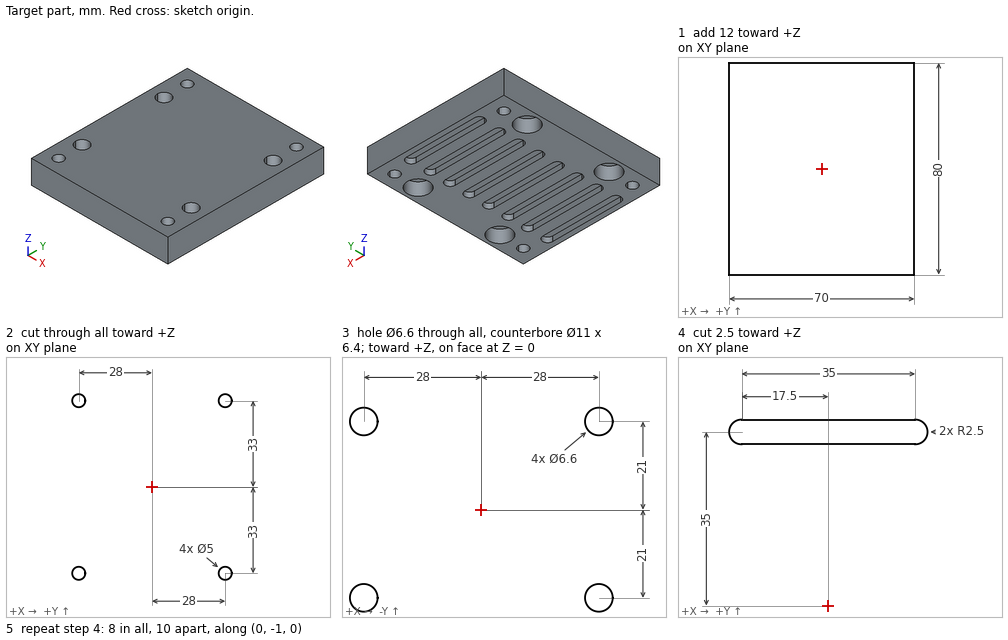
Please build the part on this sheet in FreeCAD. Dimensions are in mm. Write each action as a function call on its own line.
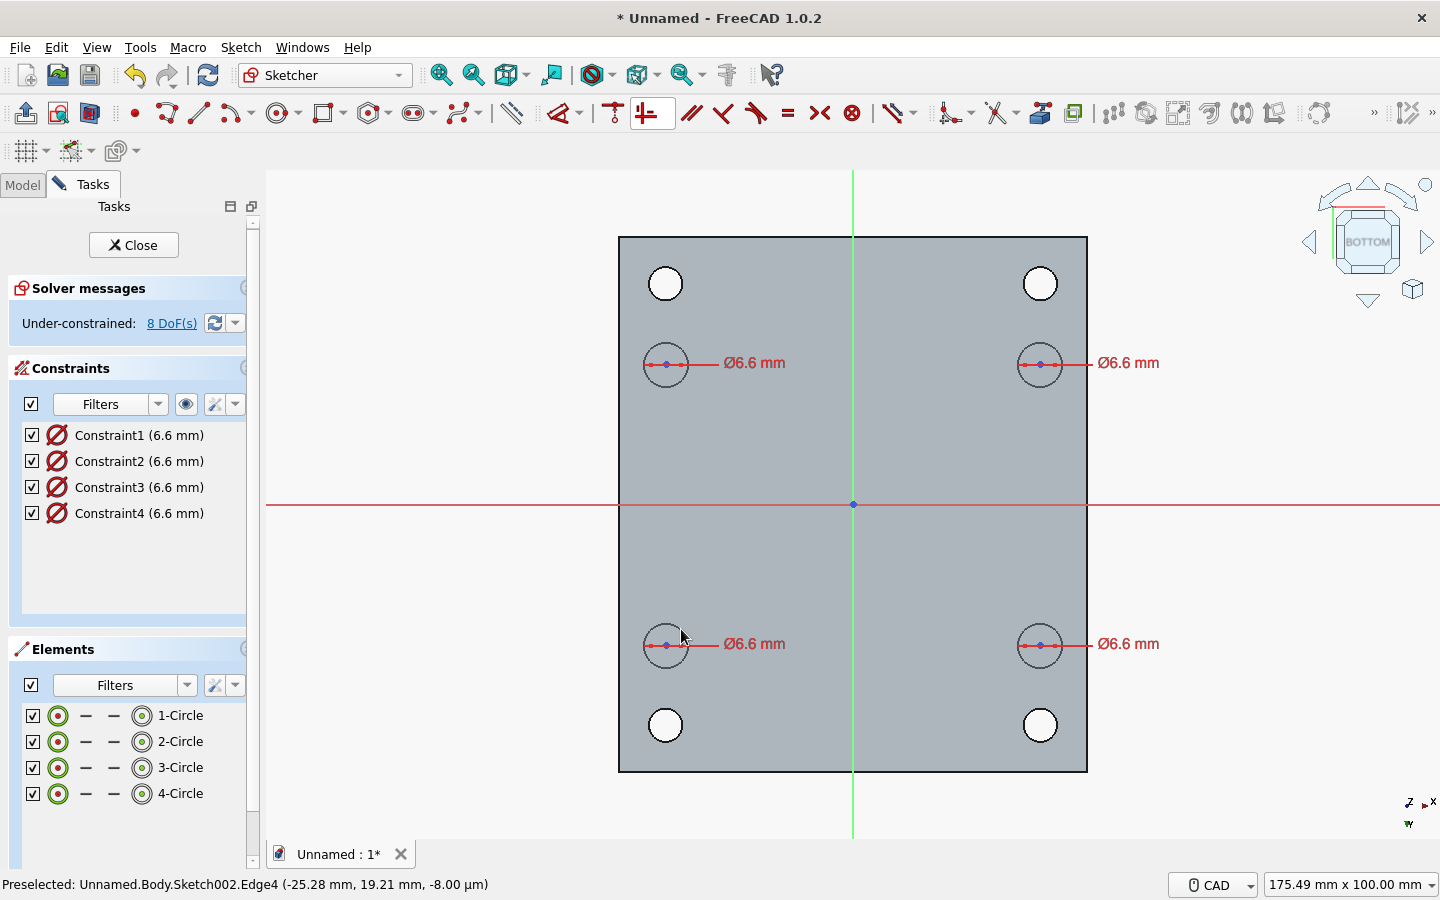
click(1040, 365)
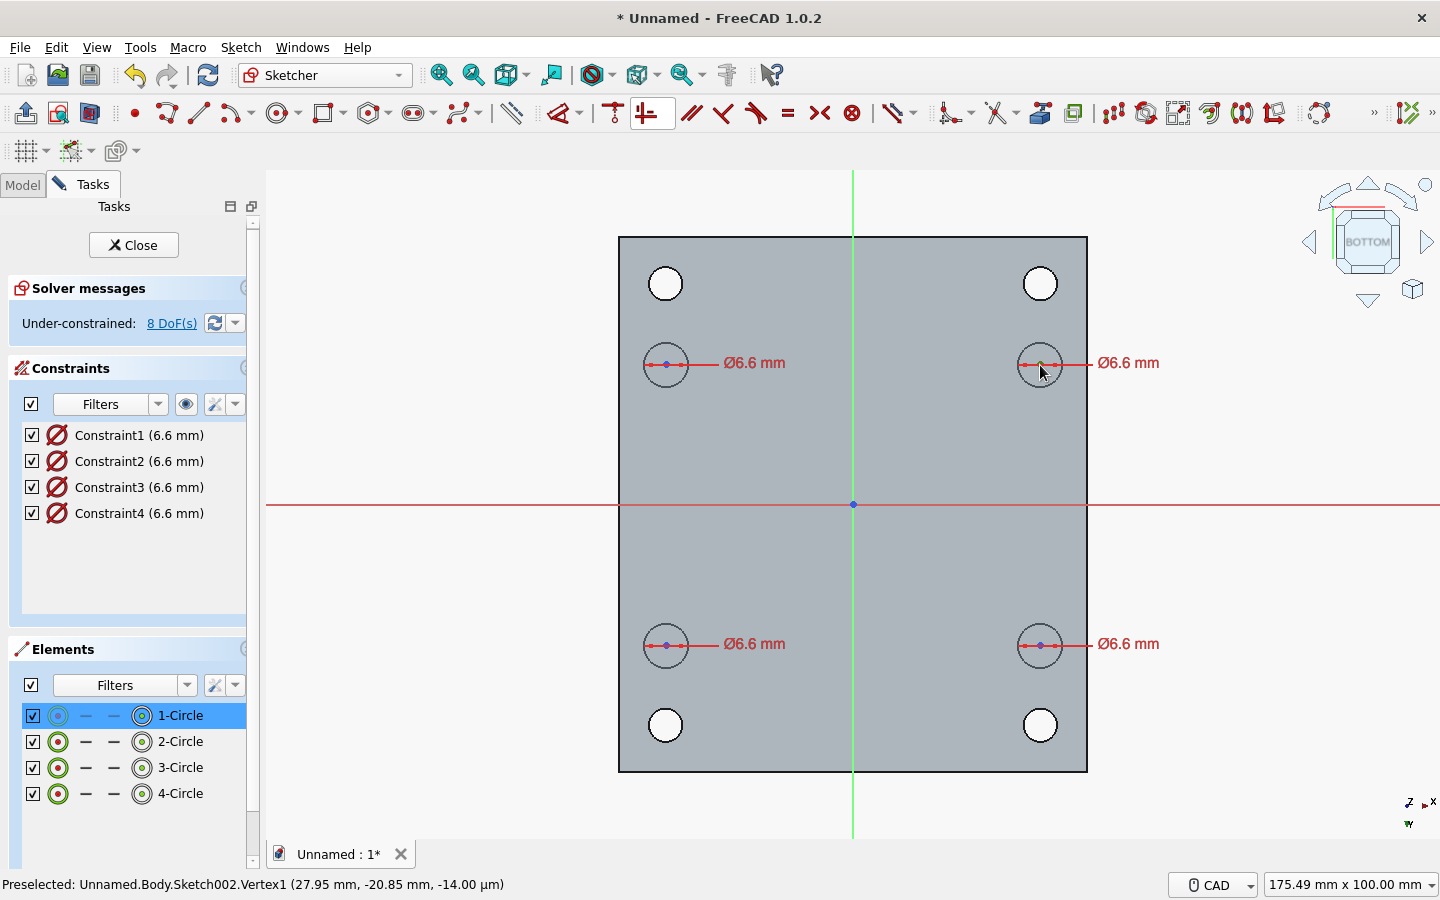
click(1040, 646)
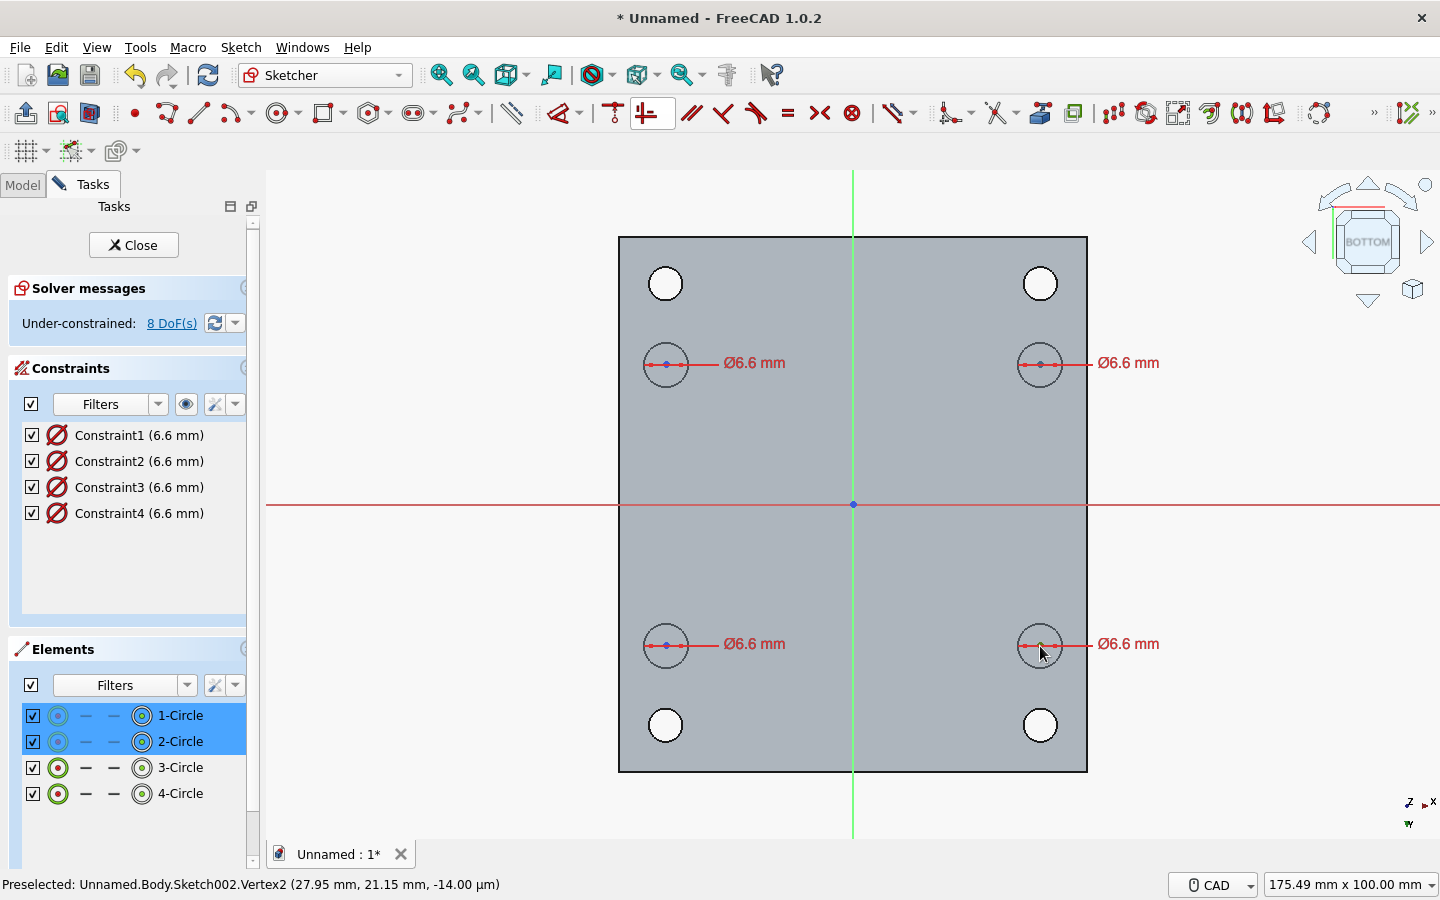
key(v)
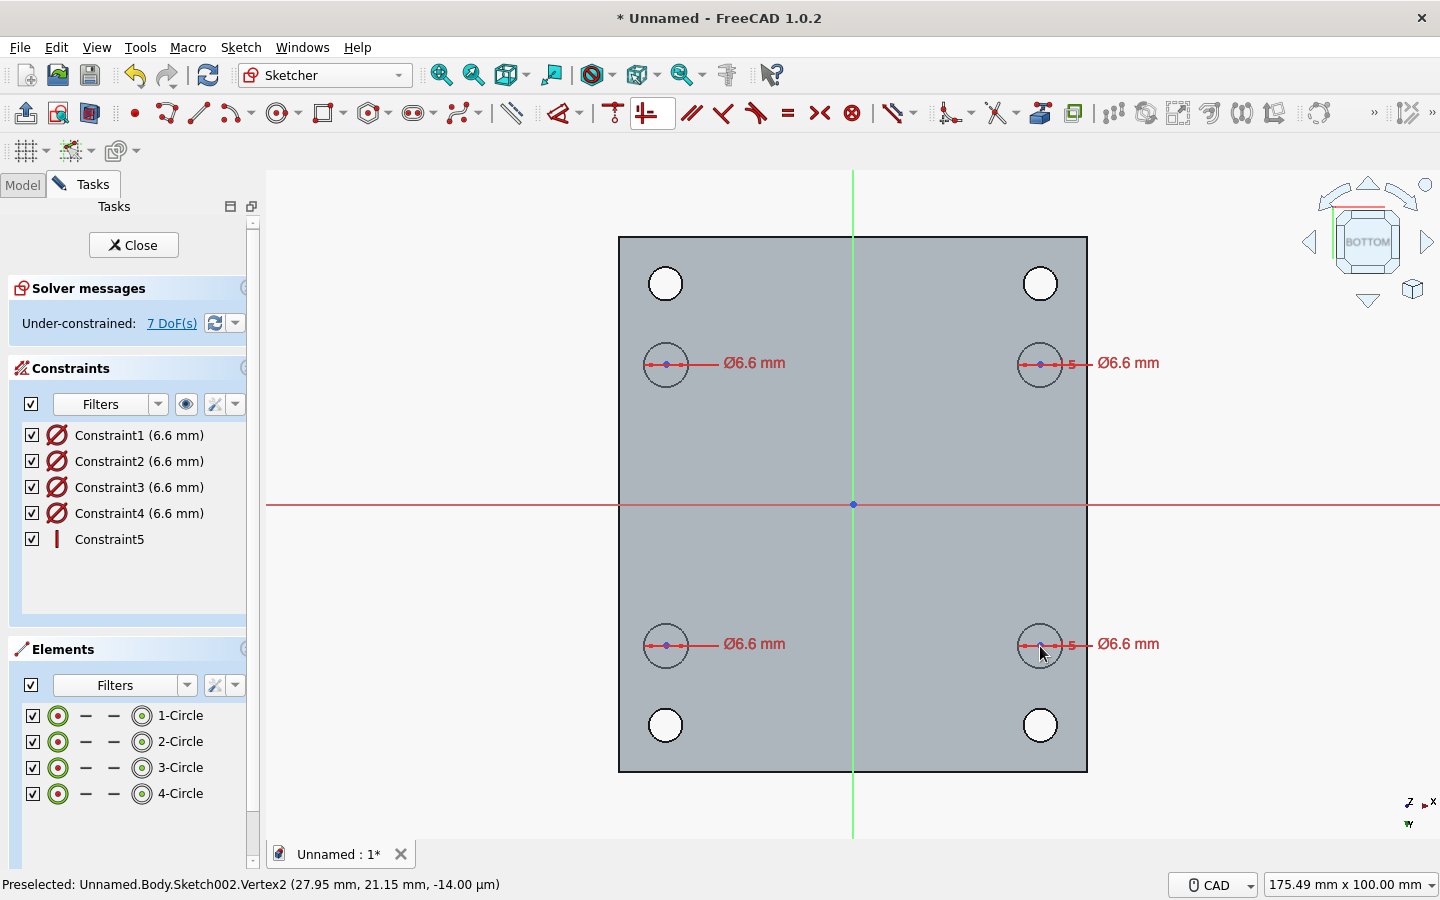
click(1040, 365)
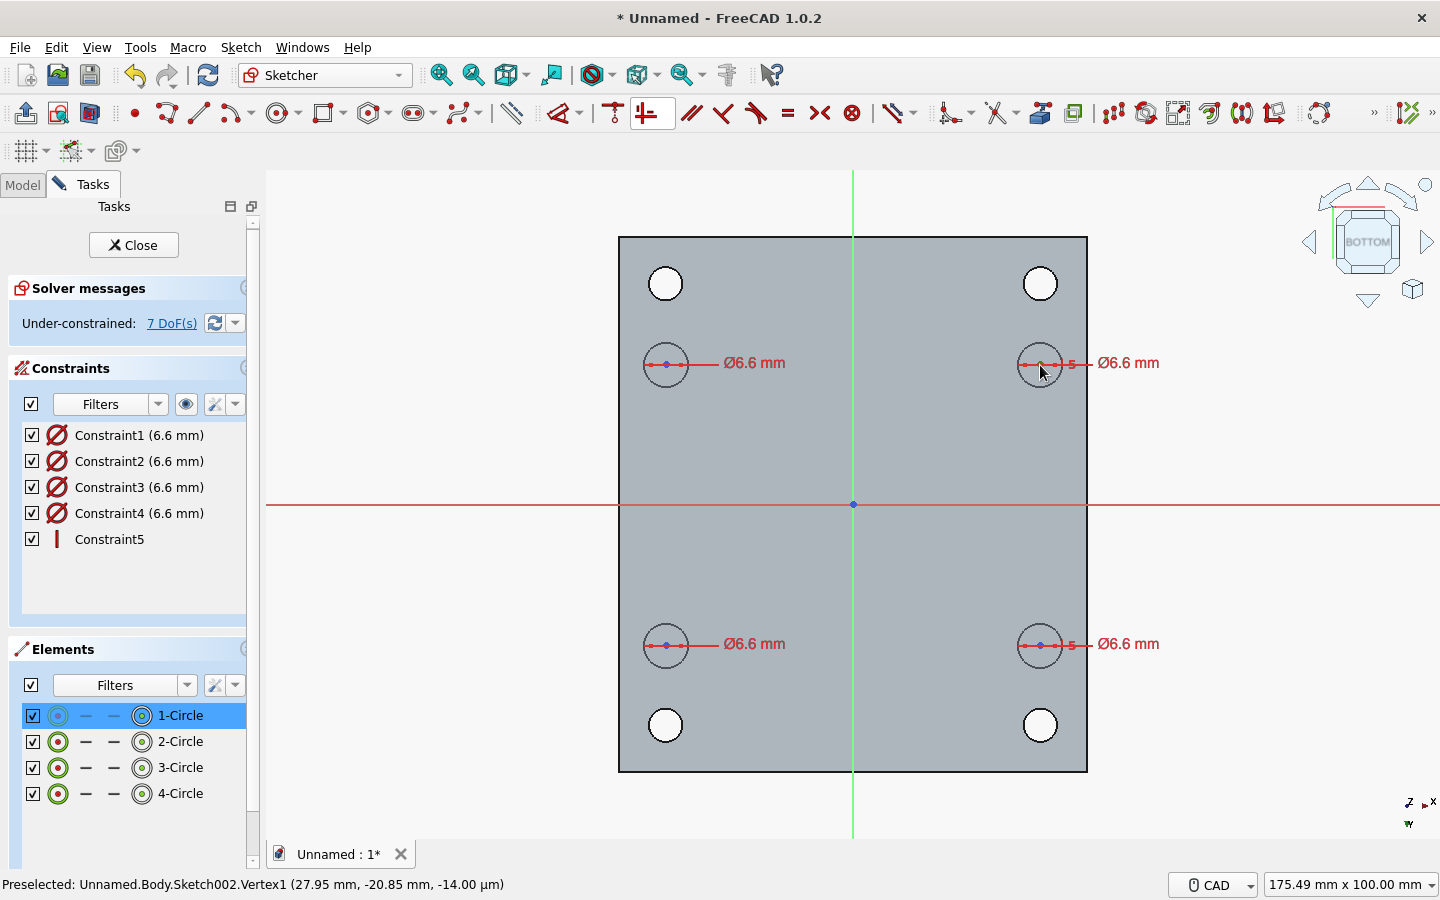
click(666, 365)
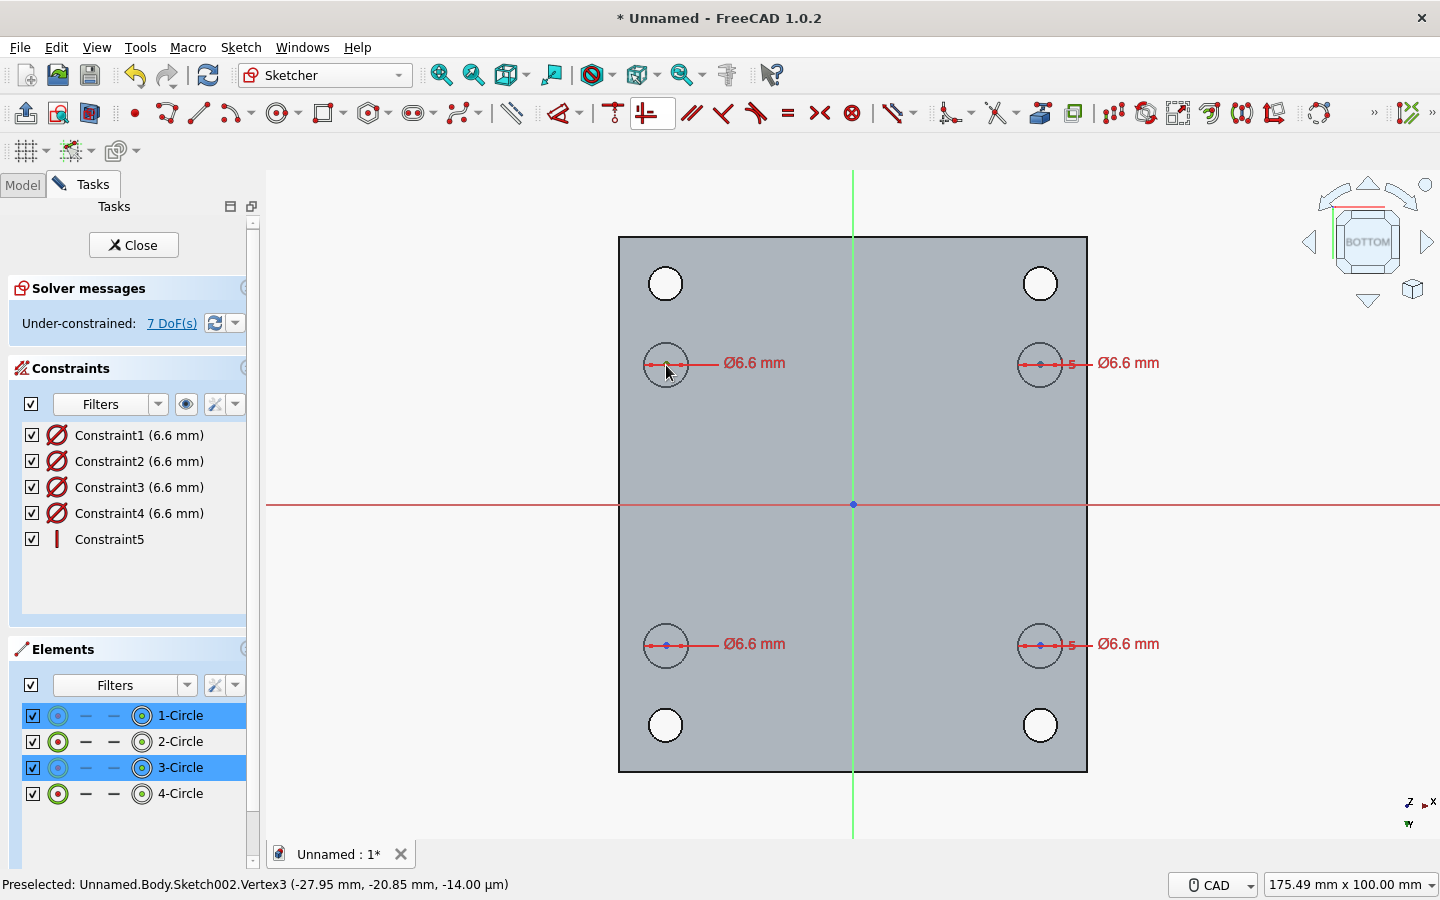
click(670, 114)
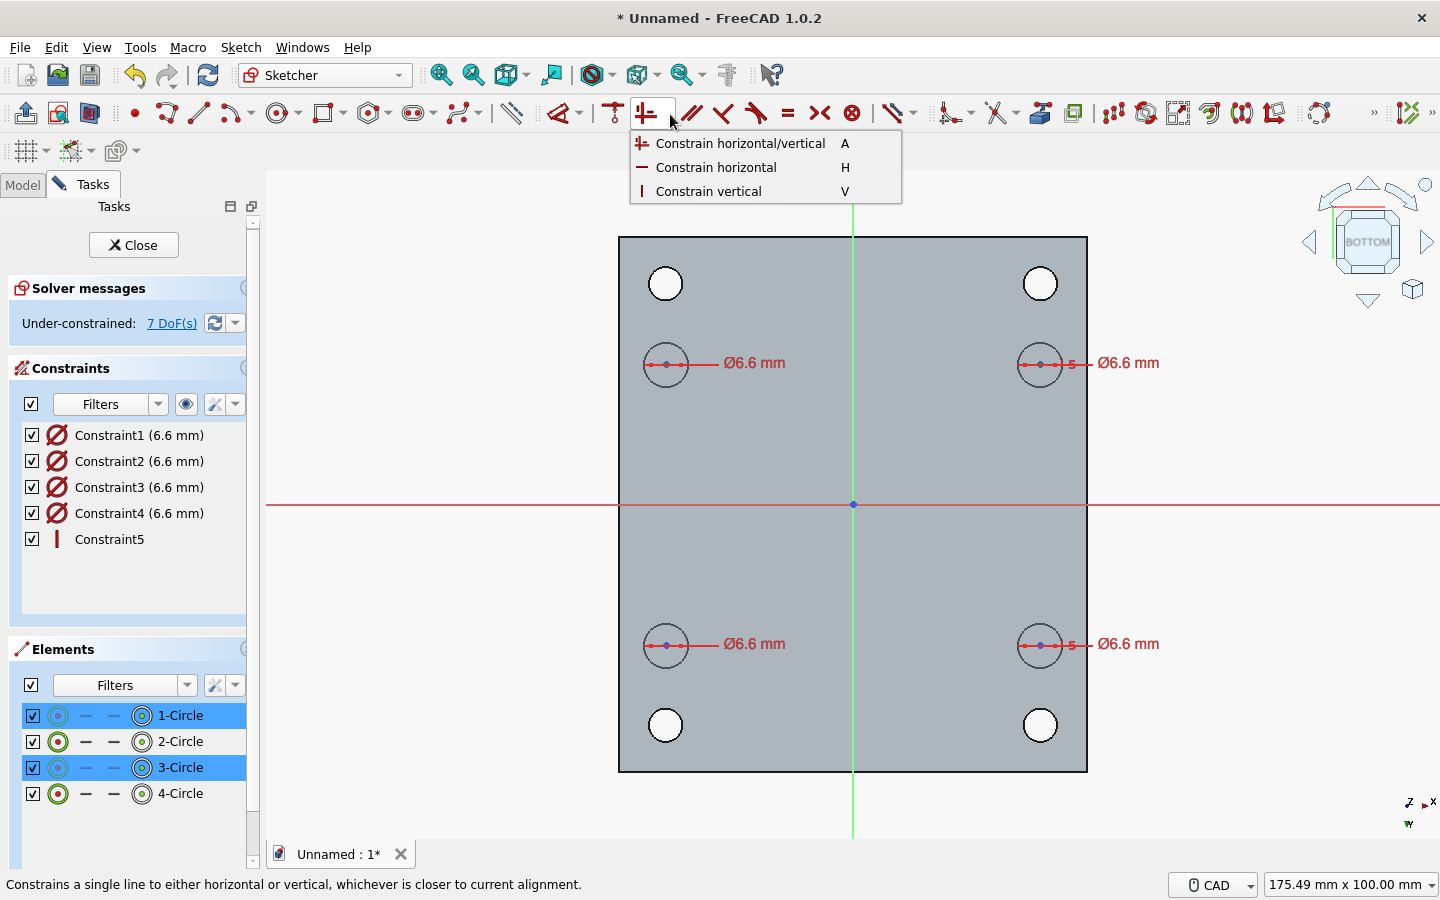
click(766, 167)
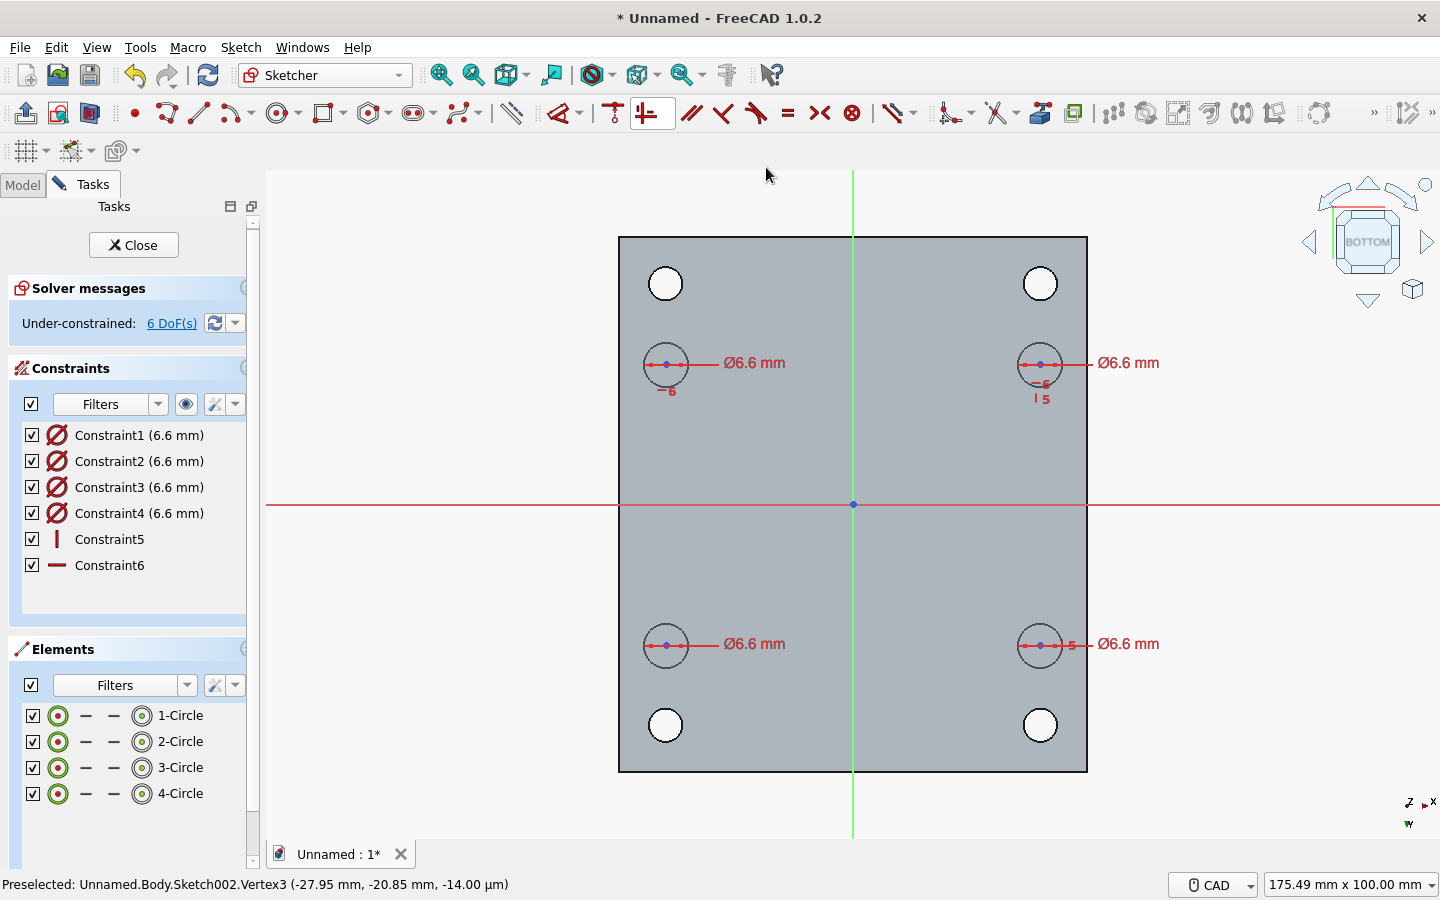
click(666, 365)